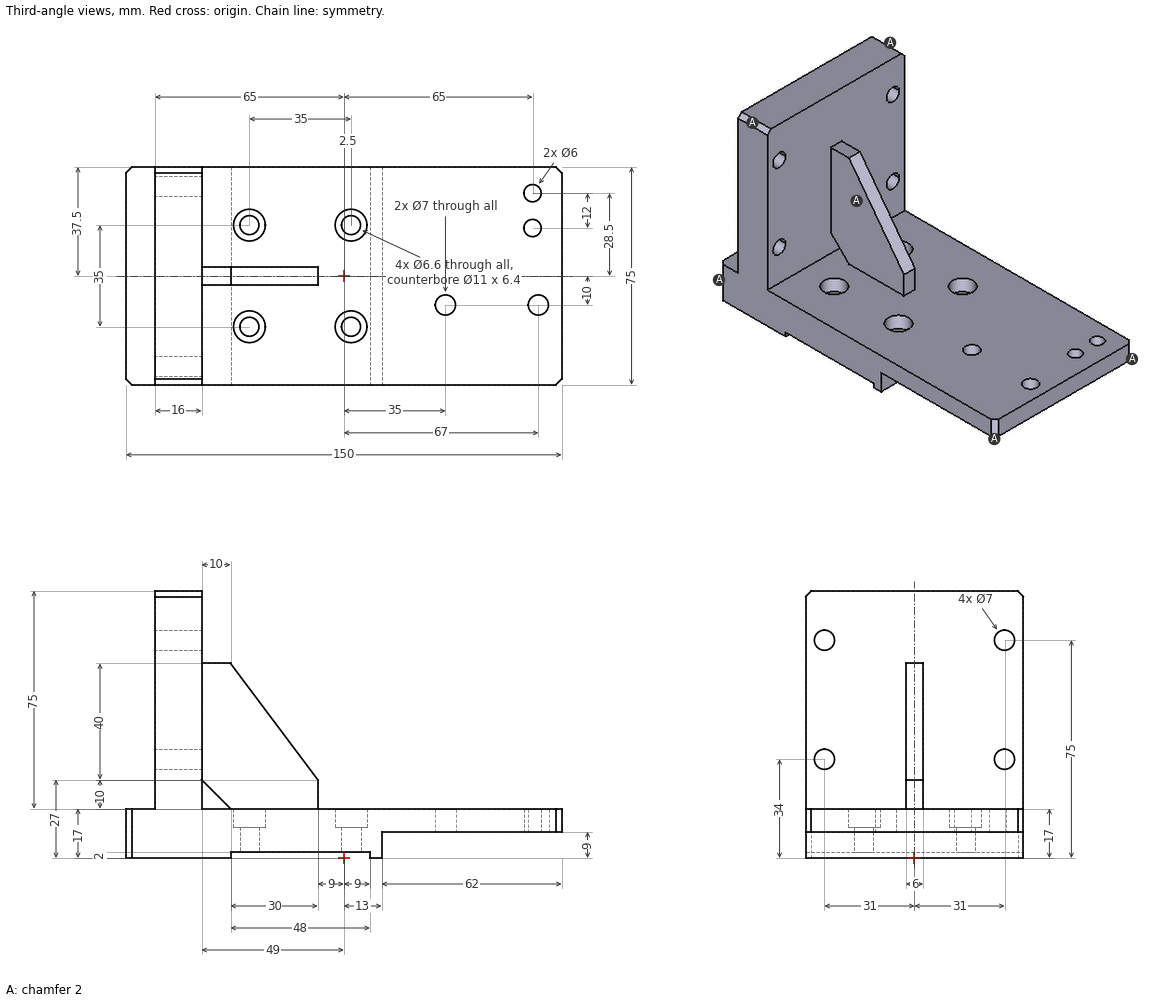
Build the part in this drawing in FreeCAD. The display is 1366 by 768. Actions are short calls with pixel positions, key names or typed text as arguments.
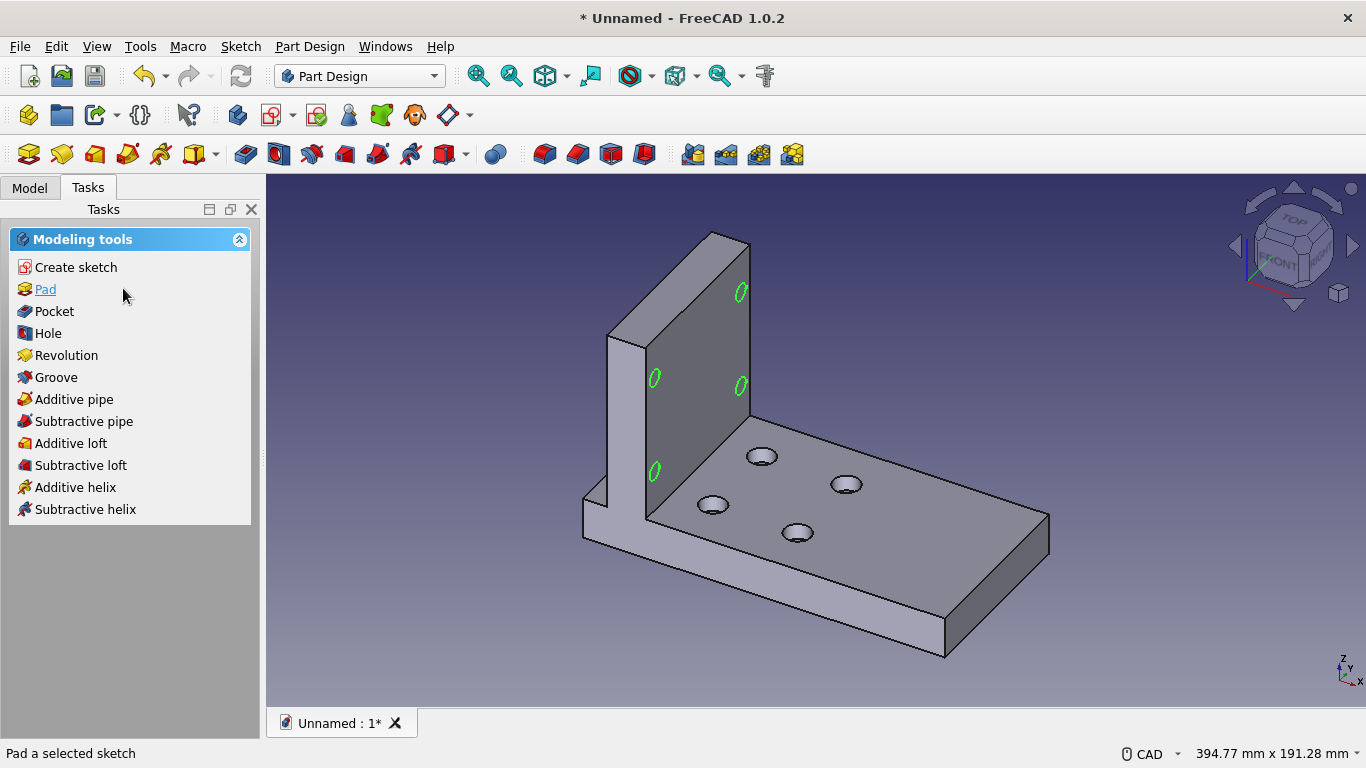
click(246, 154)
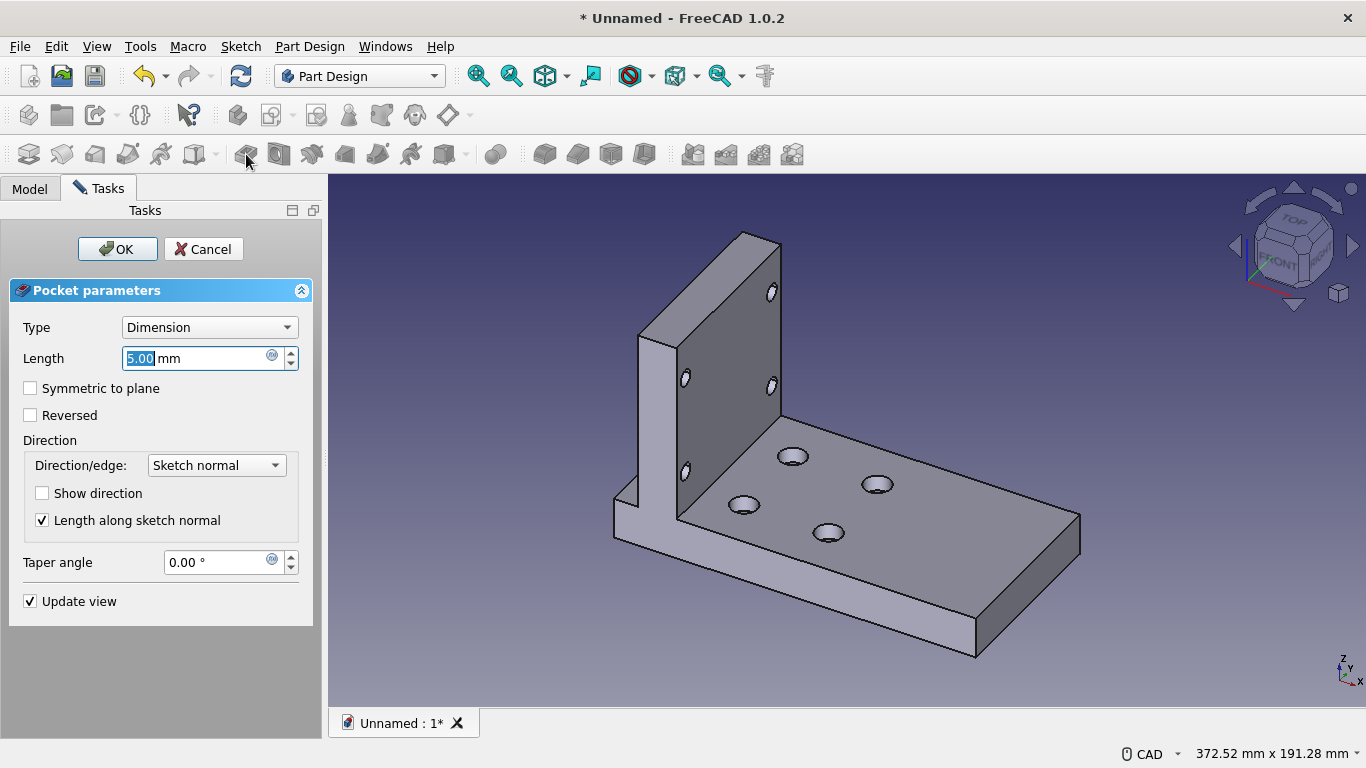
click(210, 328)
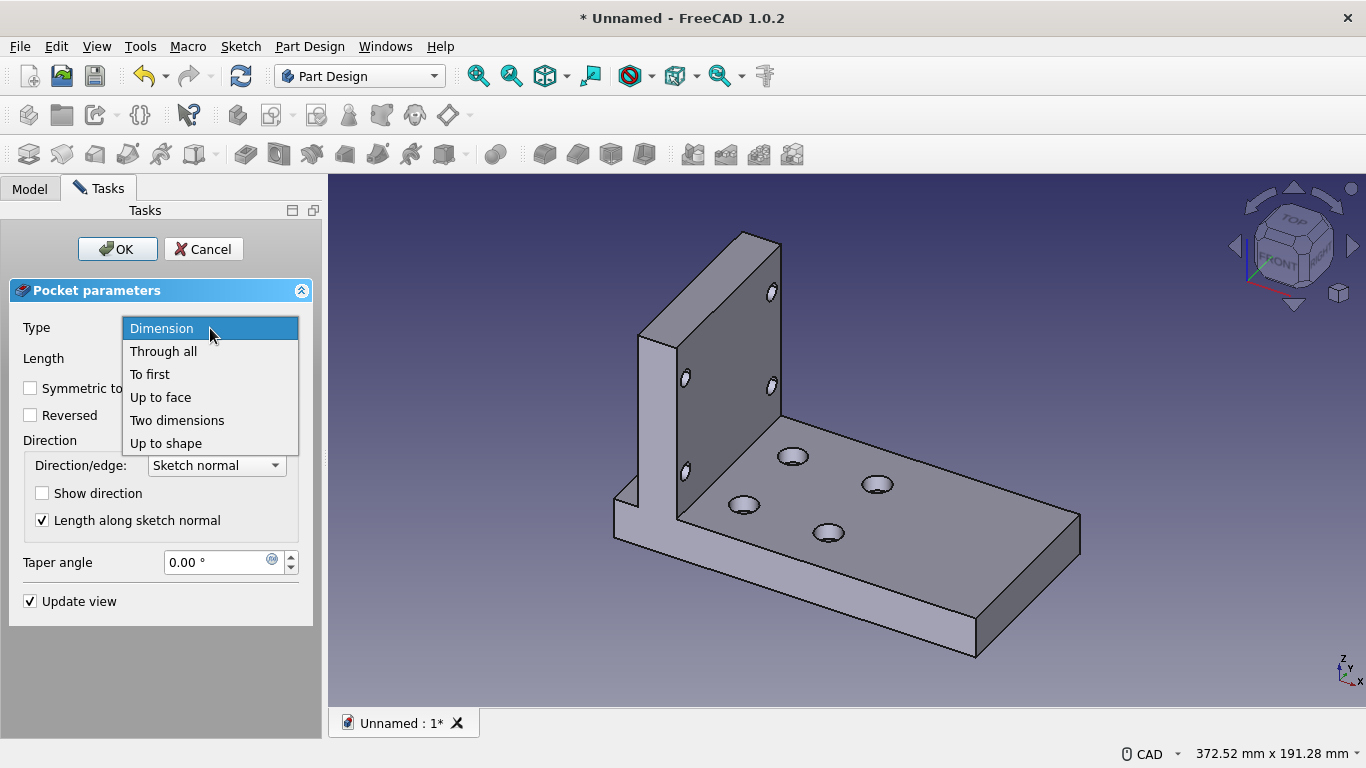
click(208, 352)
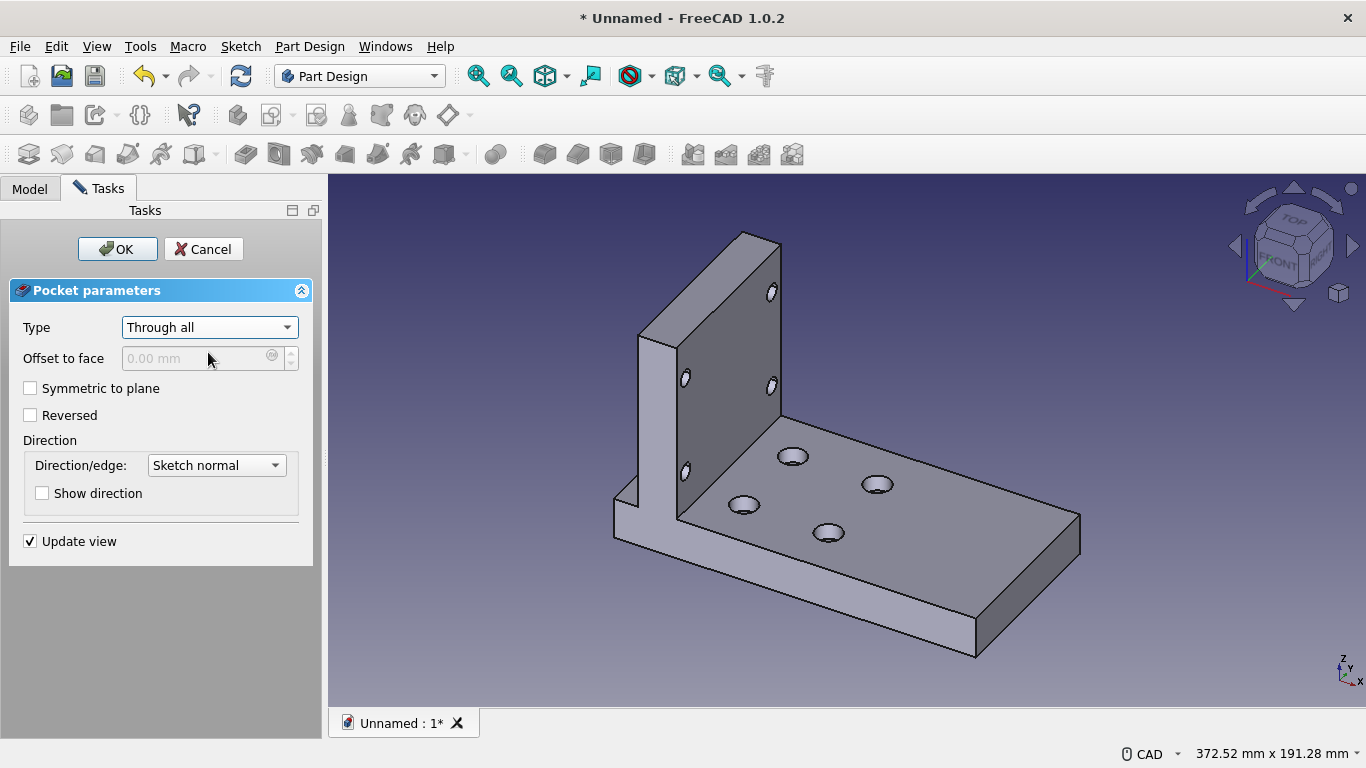
click(118, 249)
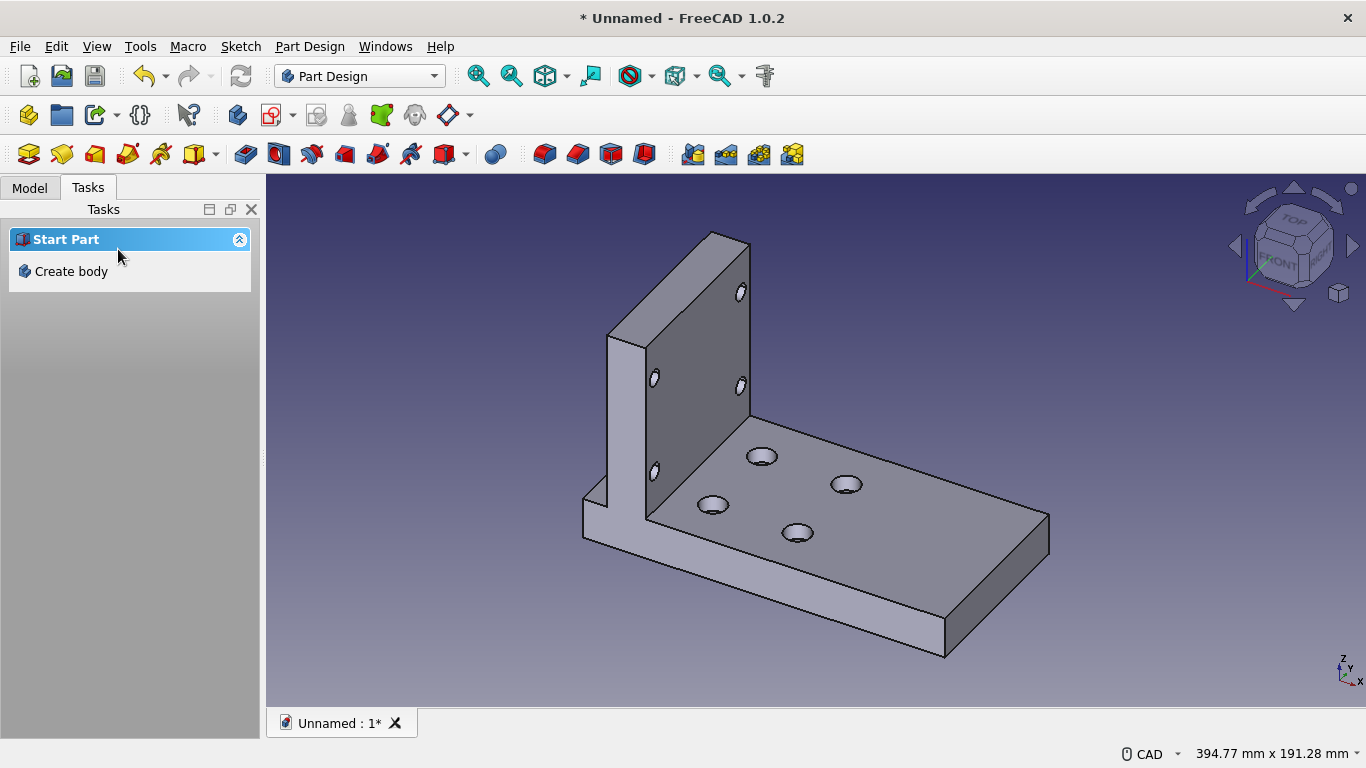
click(919, 633)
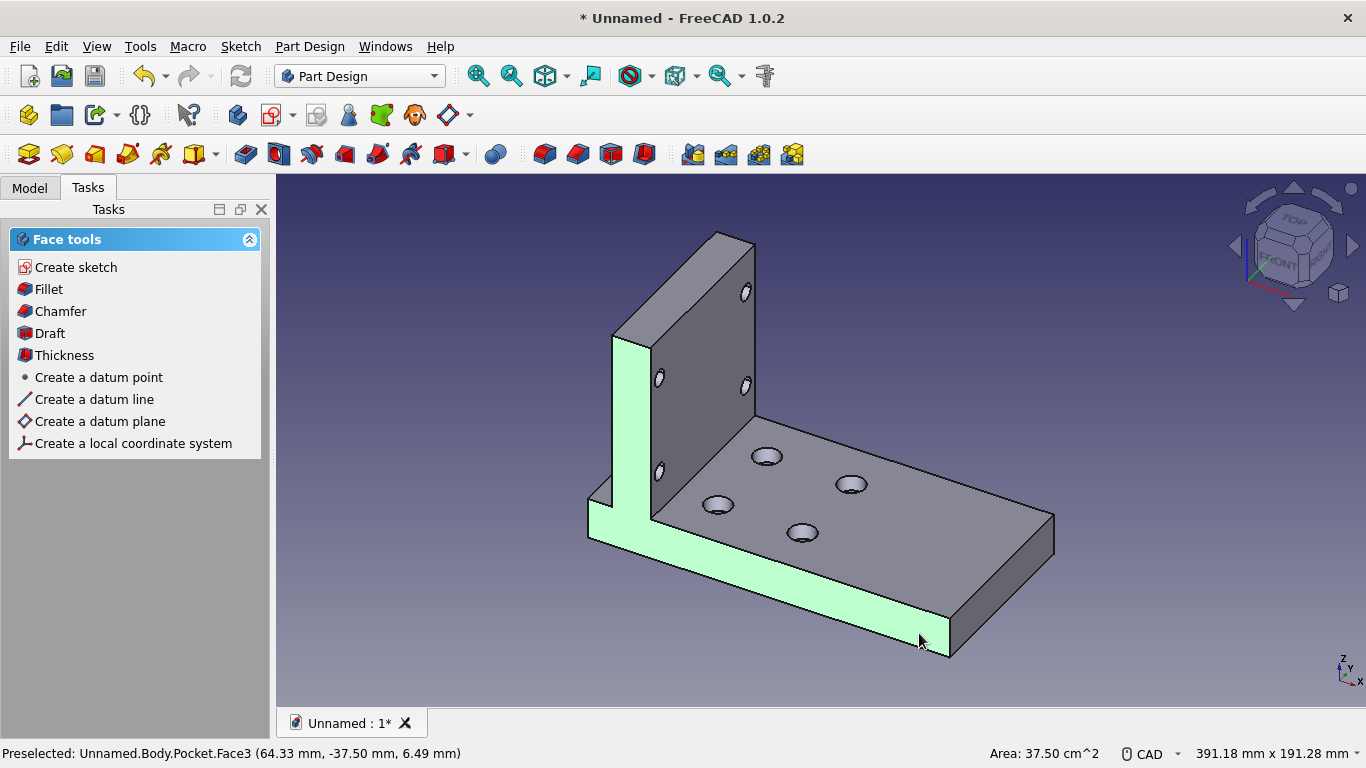
click(270, 116)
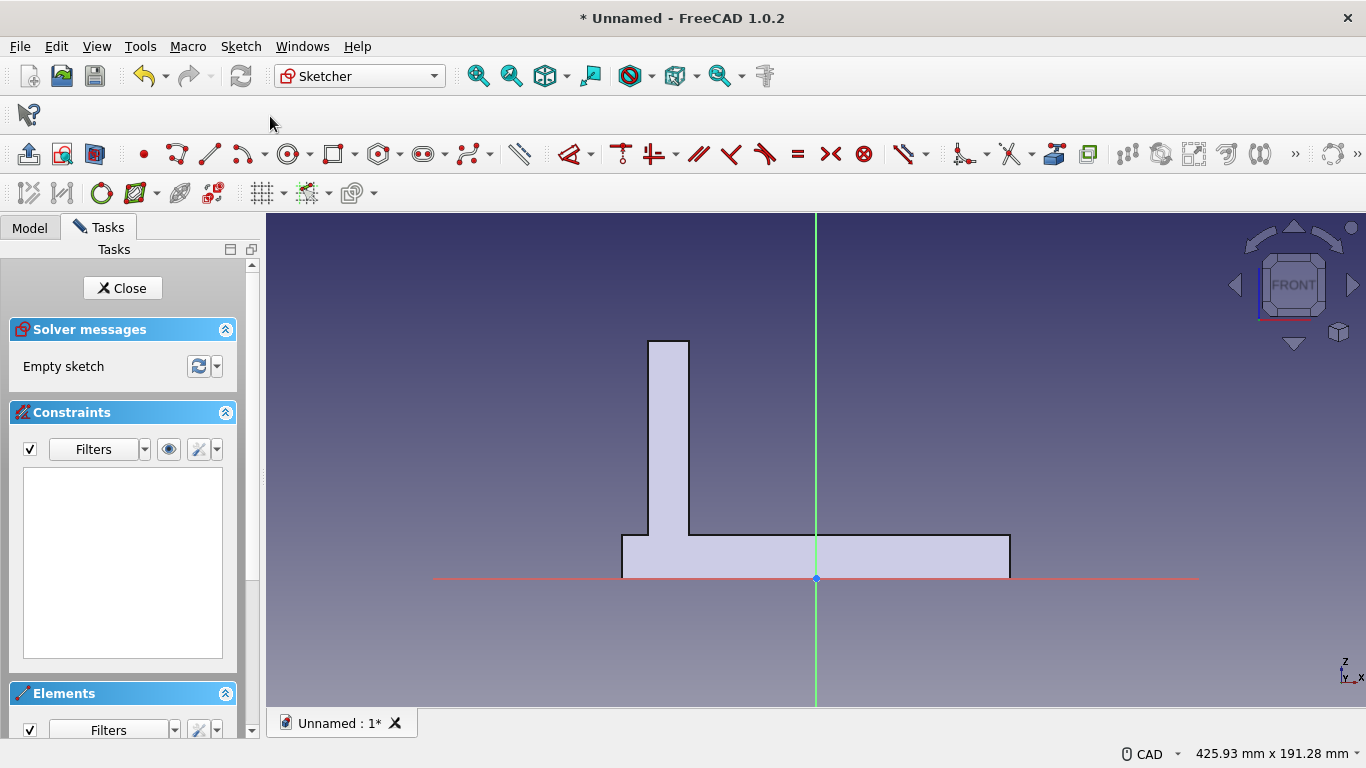
scroll(785, 606, up, 8)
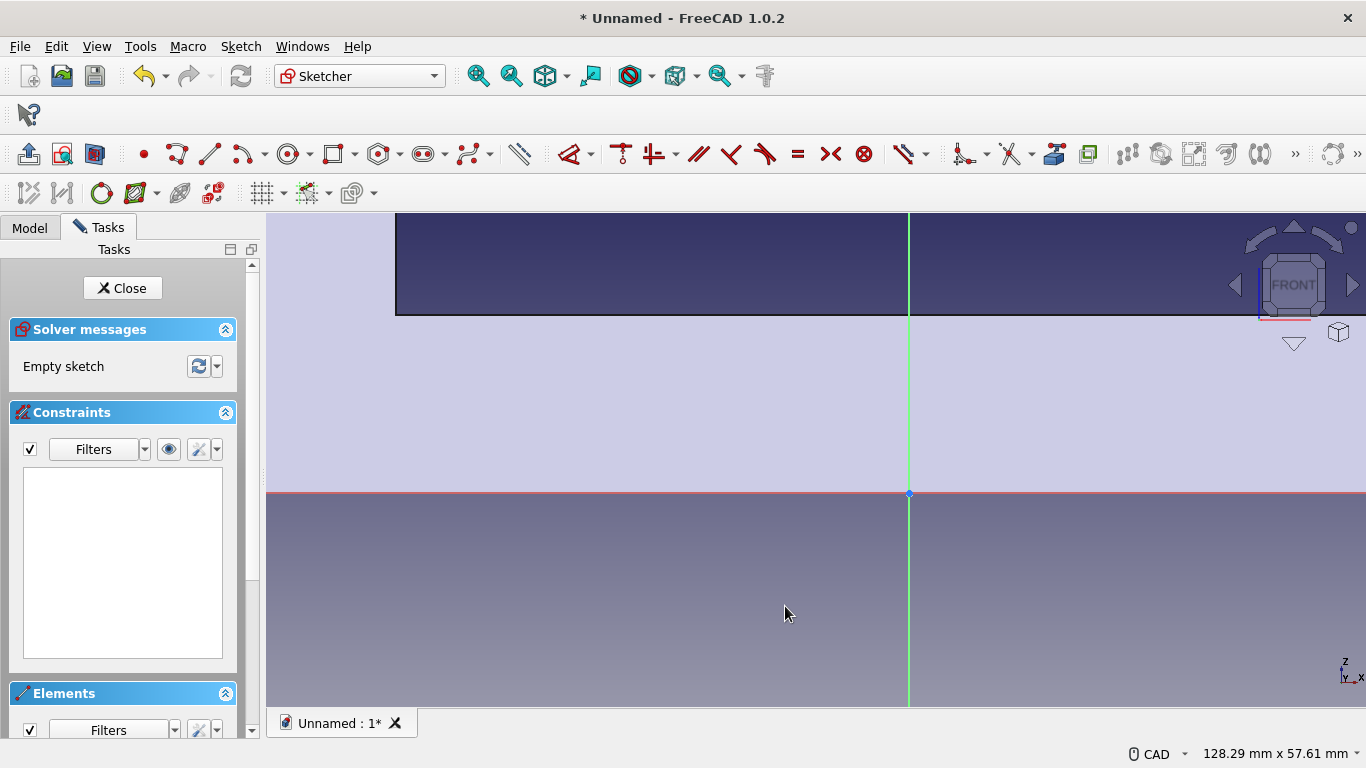
click(332, 154)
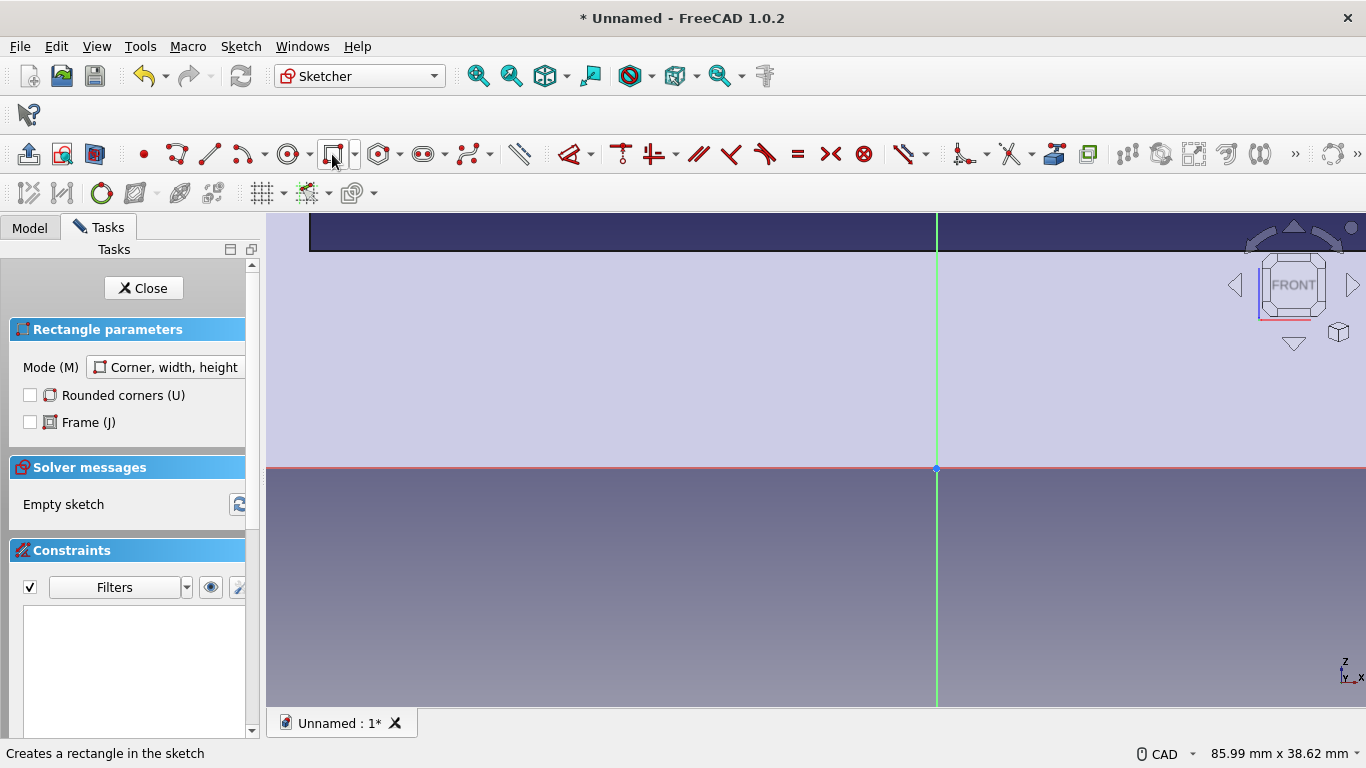
click(438, 443)
click(1052, 468)
key(Escape)